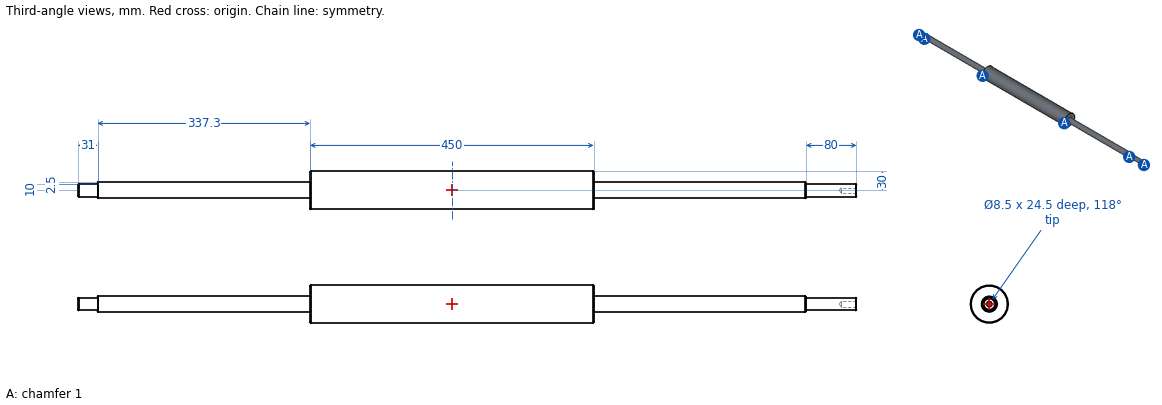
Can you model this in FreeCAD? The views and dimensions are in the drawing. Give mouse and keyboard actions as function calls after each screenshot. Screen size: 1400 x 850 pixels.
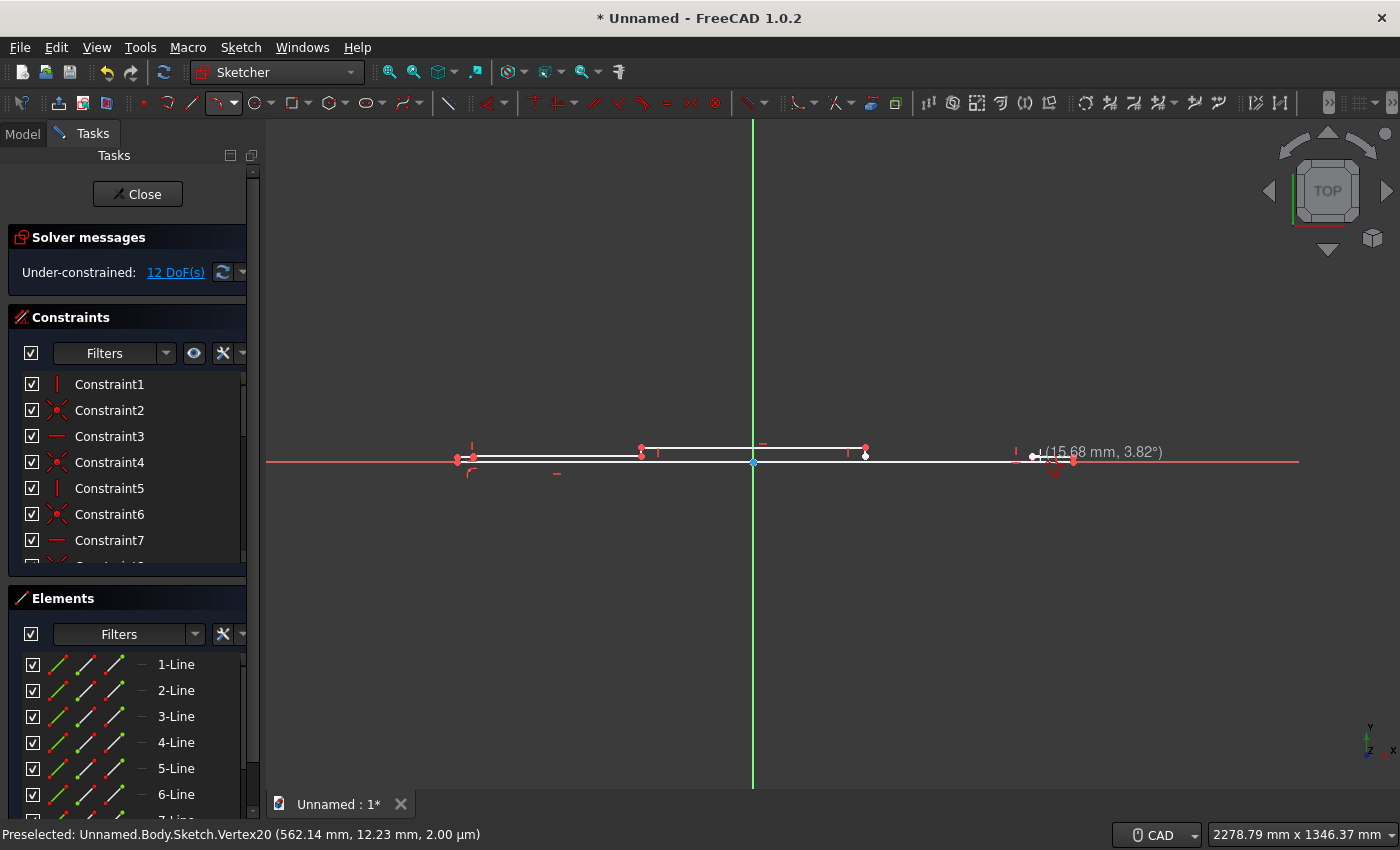
scroll(865, 456, up, 7)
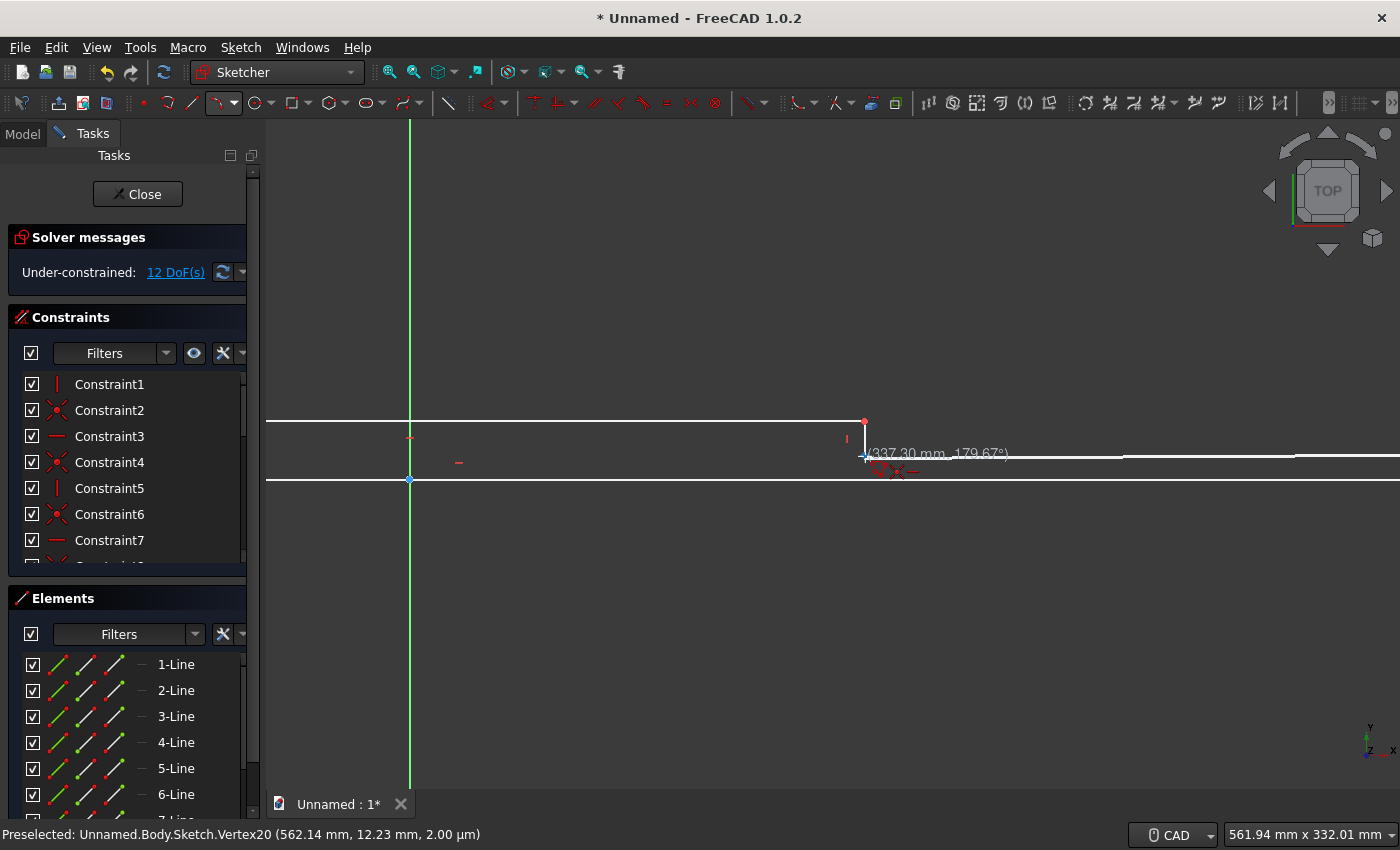
click(865, 455)
key(Escape)
key(Escape)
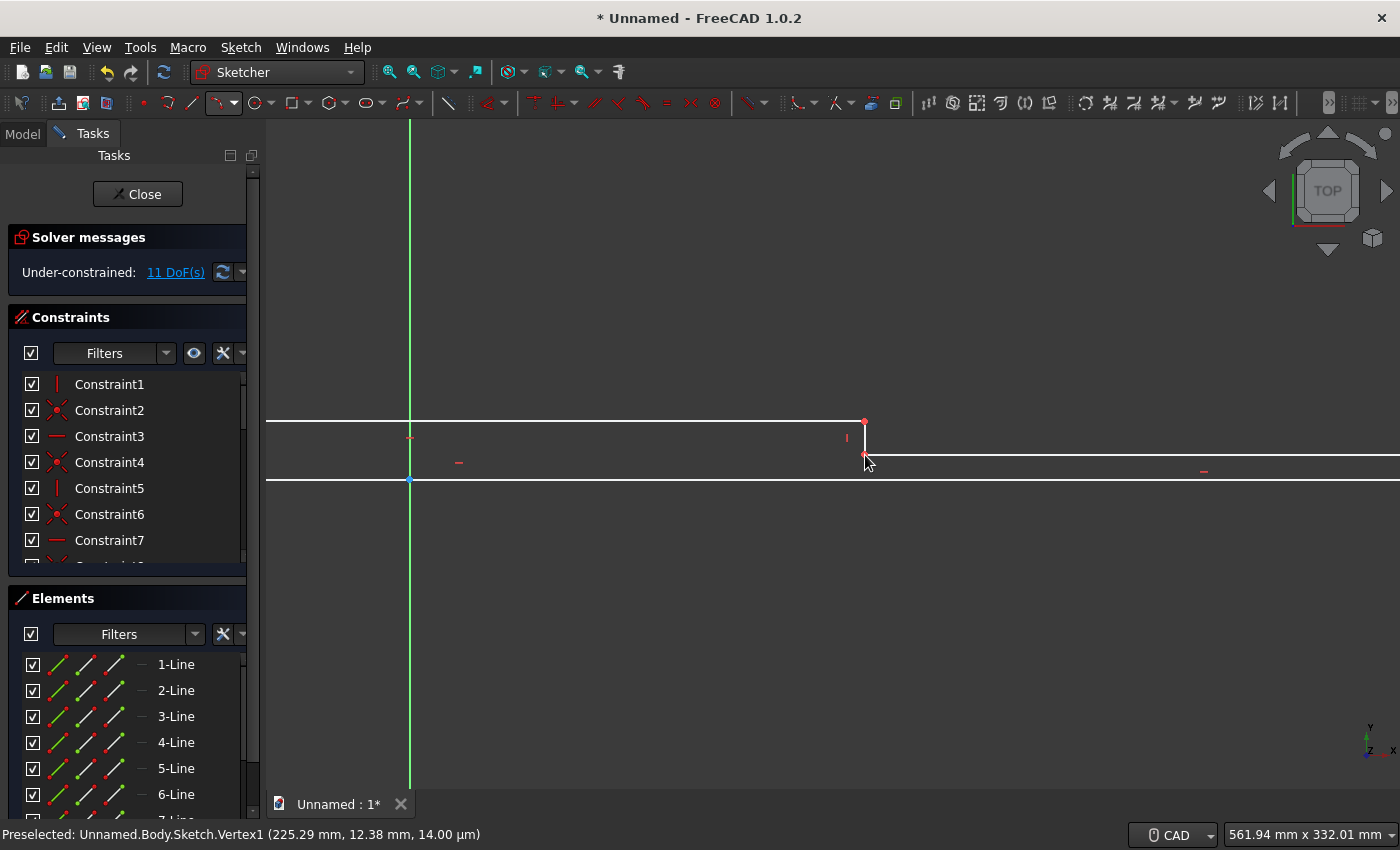
click(865, 455)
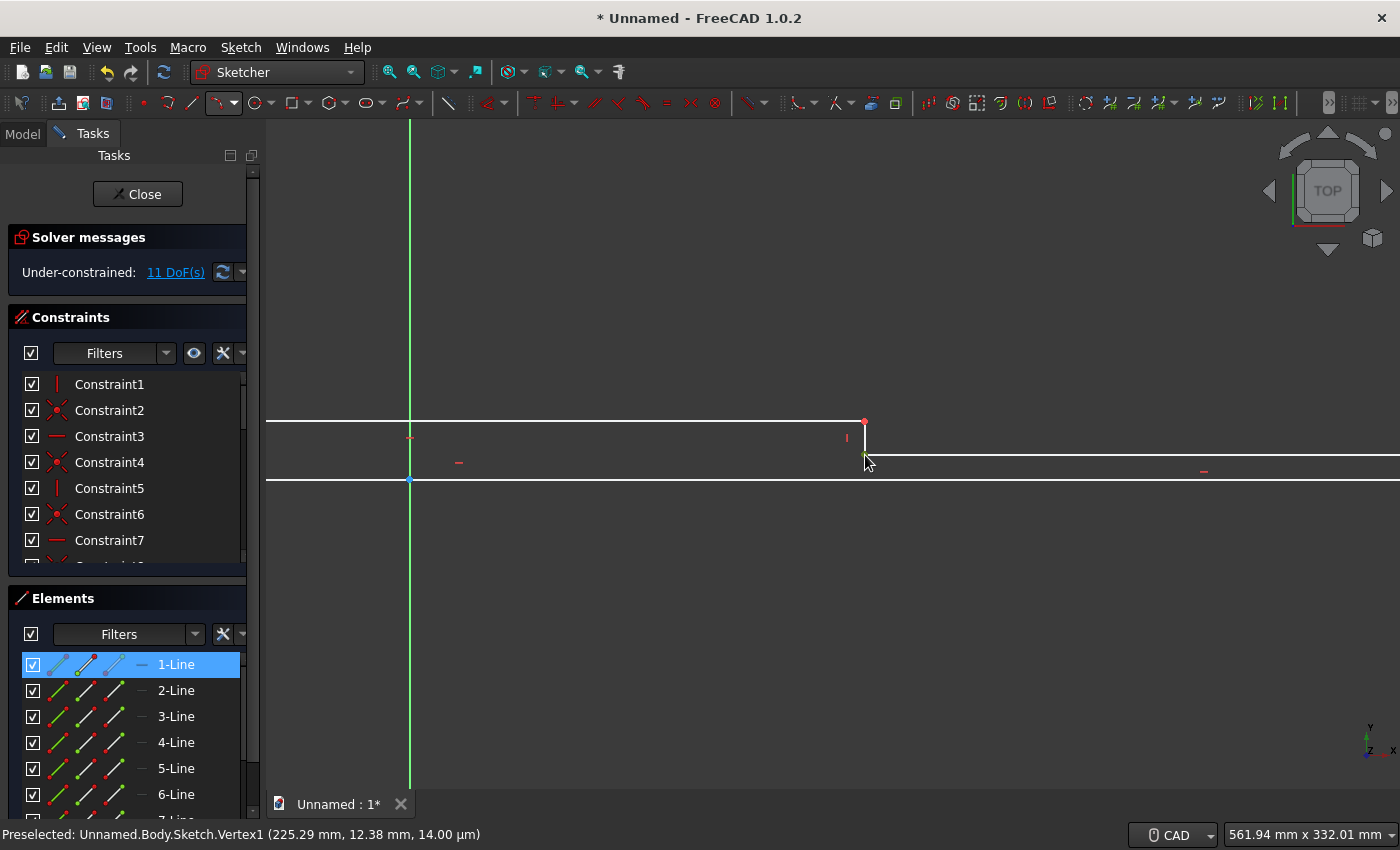
scroll(864, 456, down, 7)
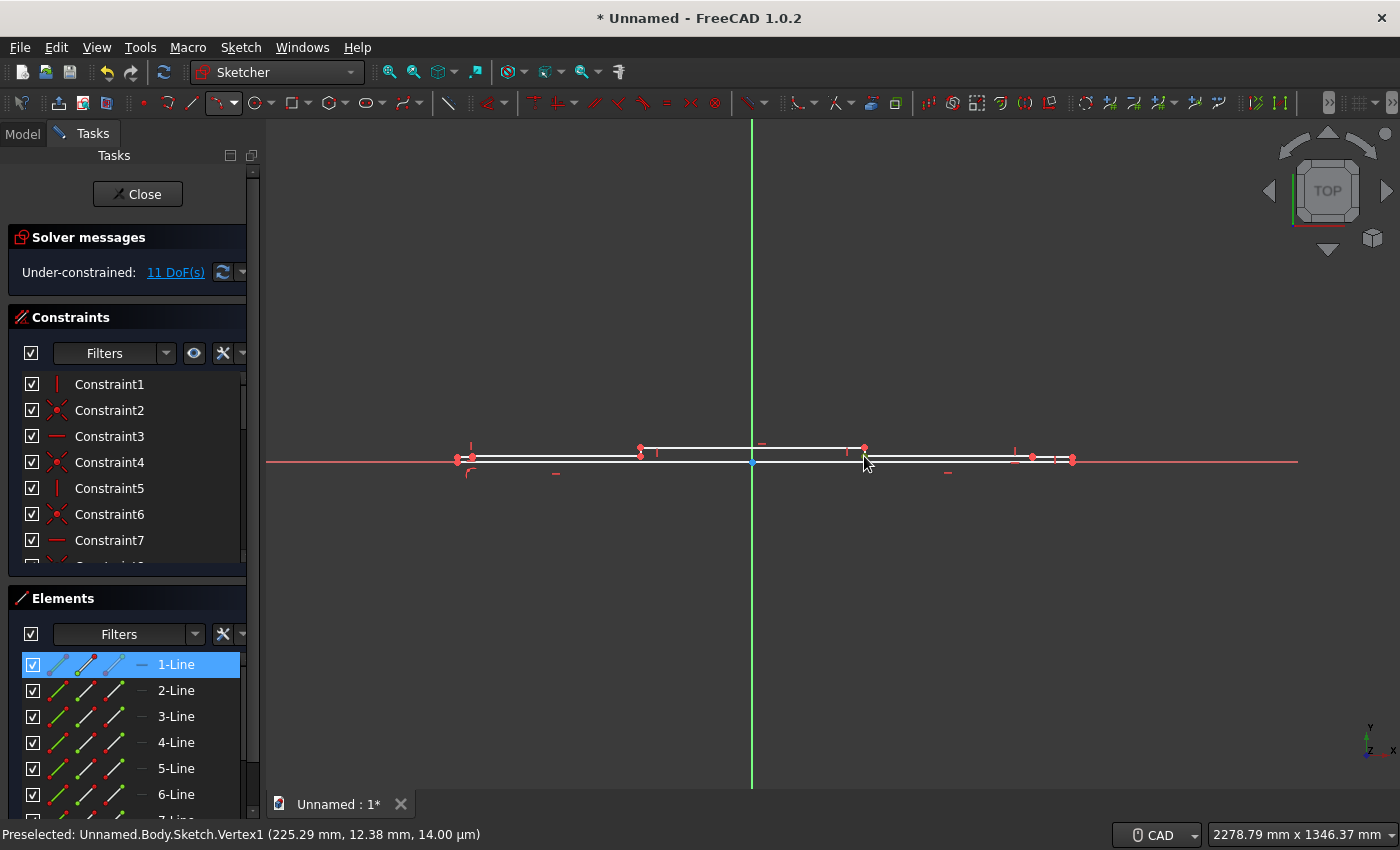
scroll(641, 456, up, 2)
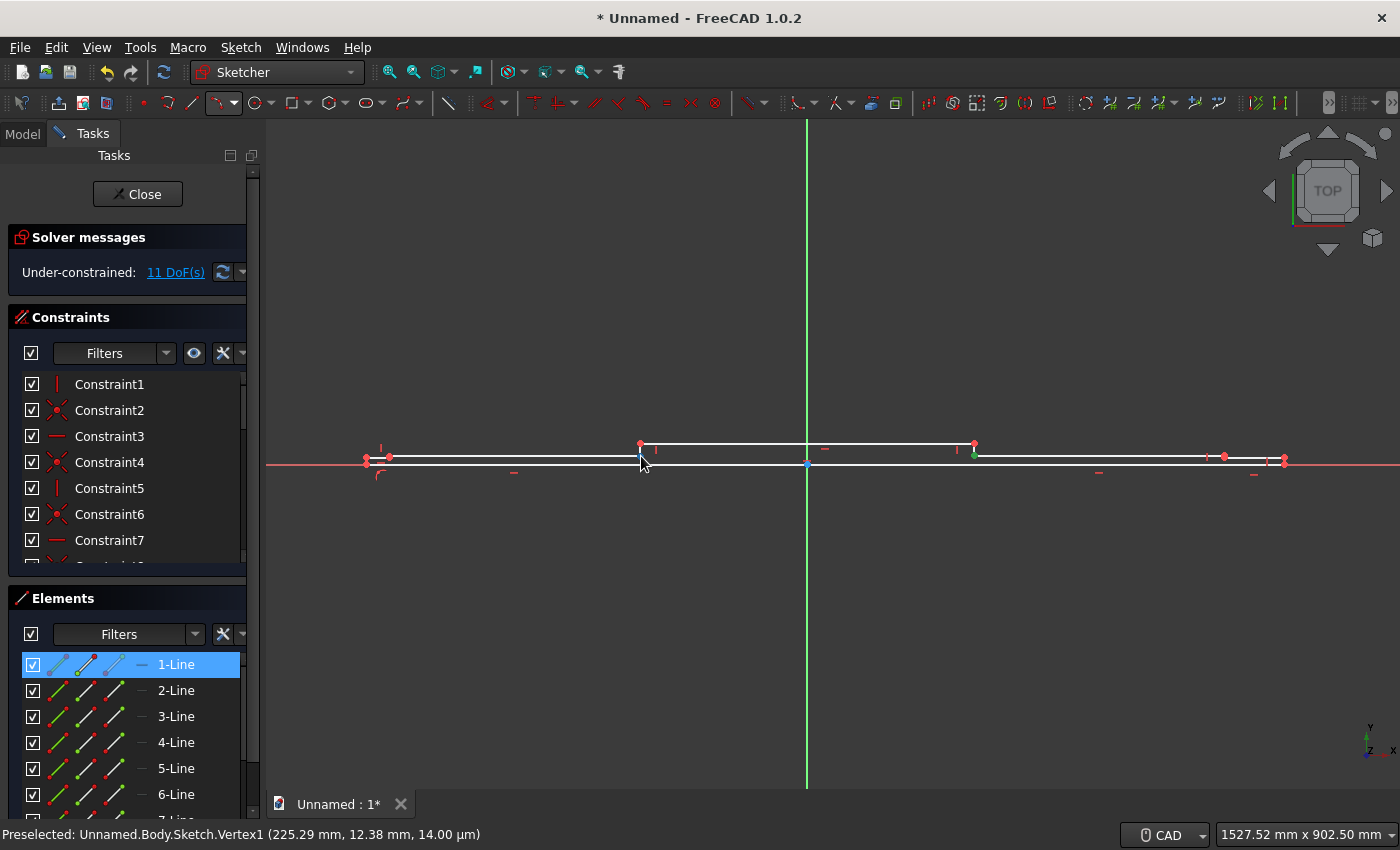
click(640, 456)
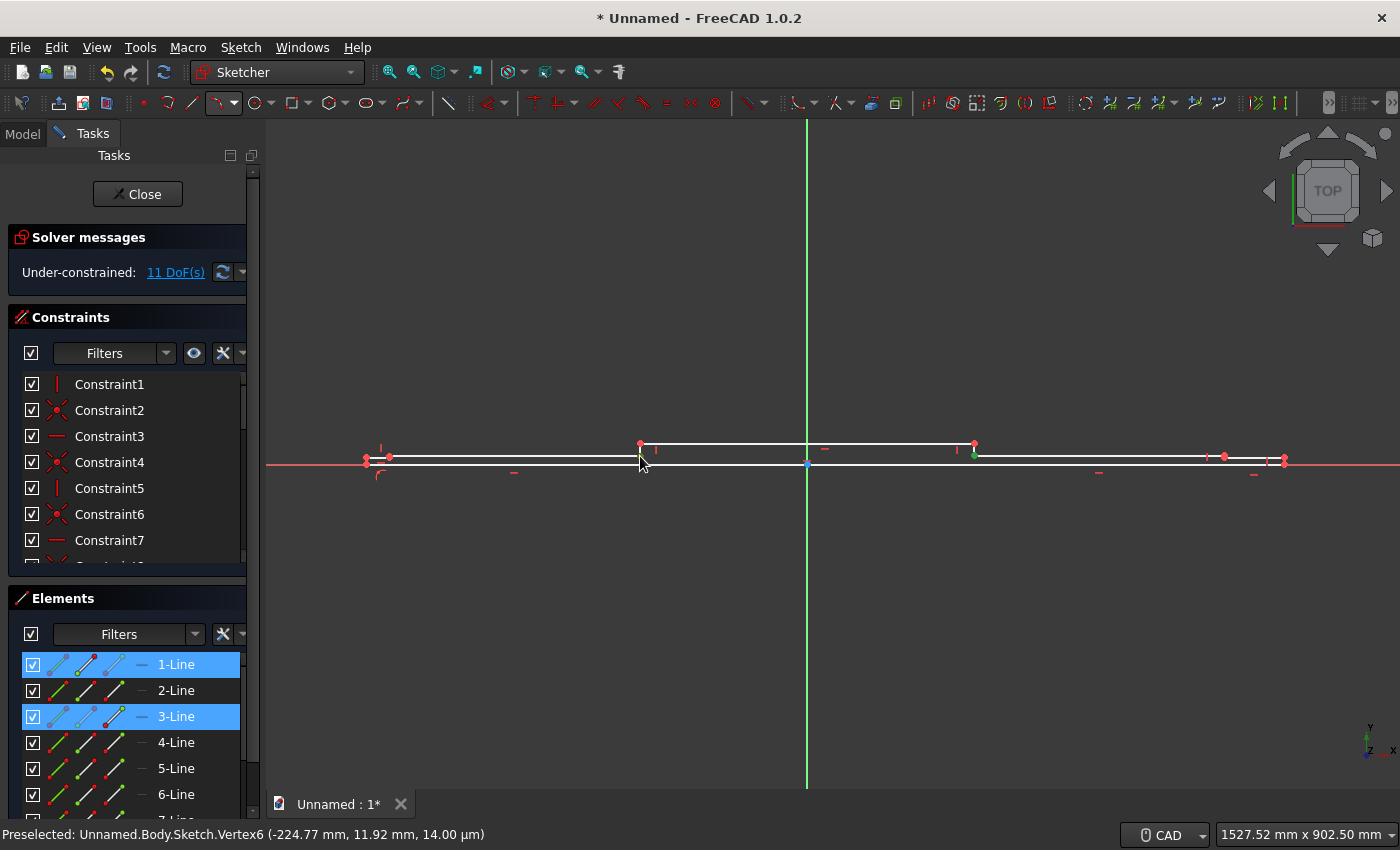
click(807, 717)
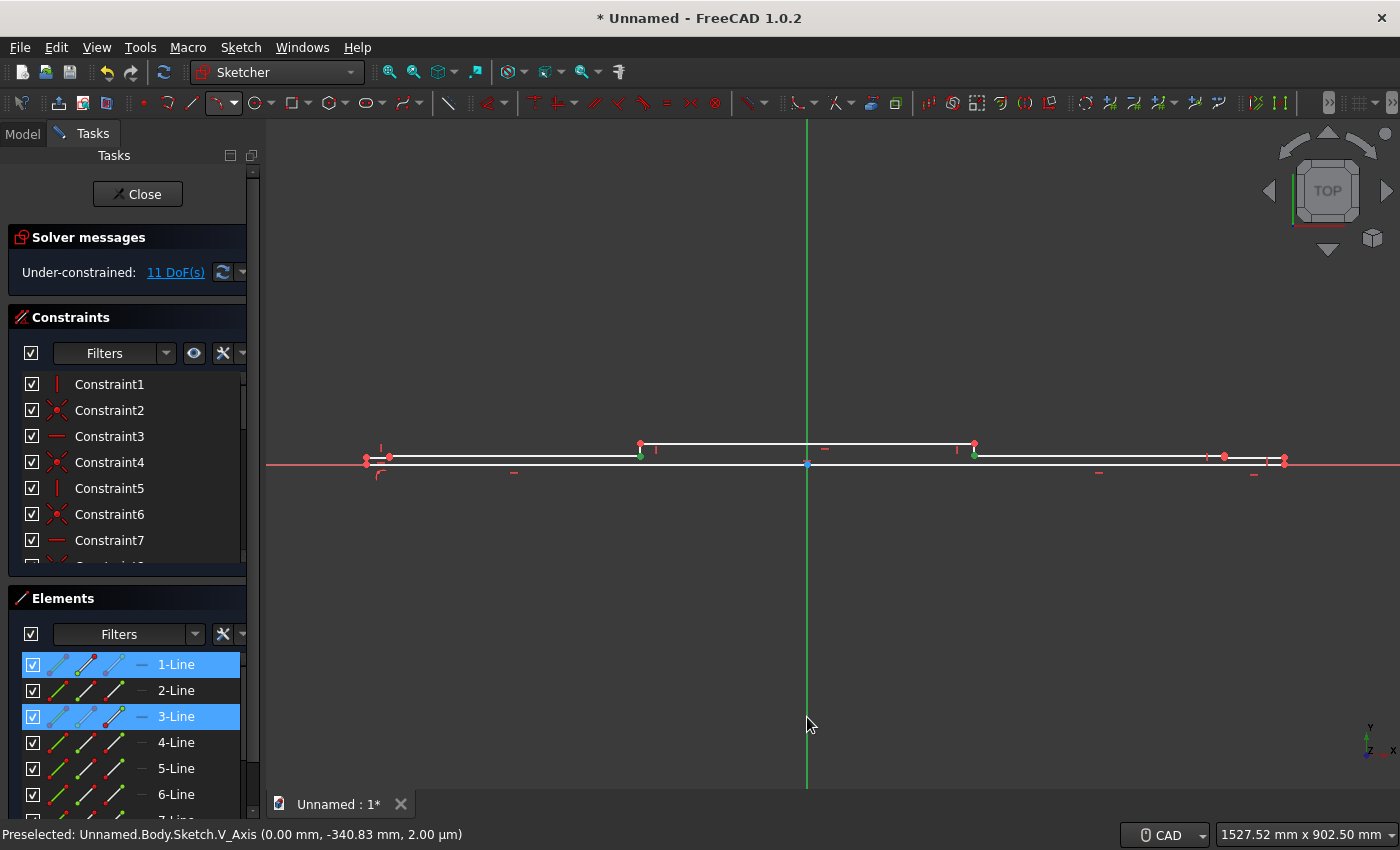
click(692, 104)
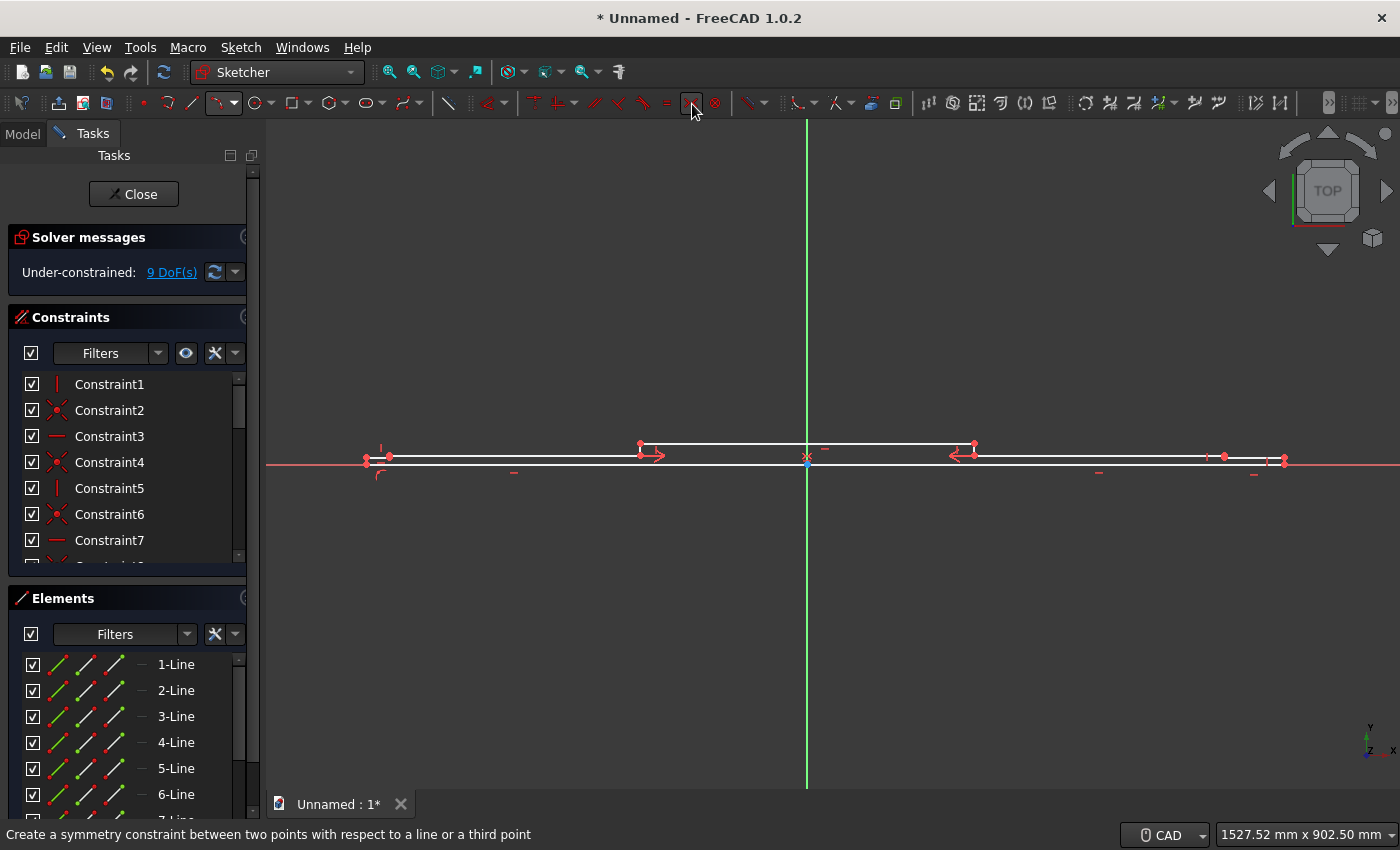
scroll(390, 458, up, 10)